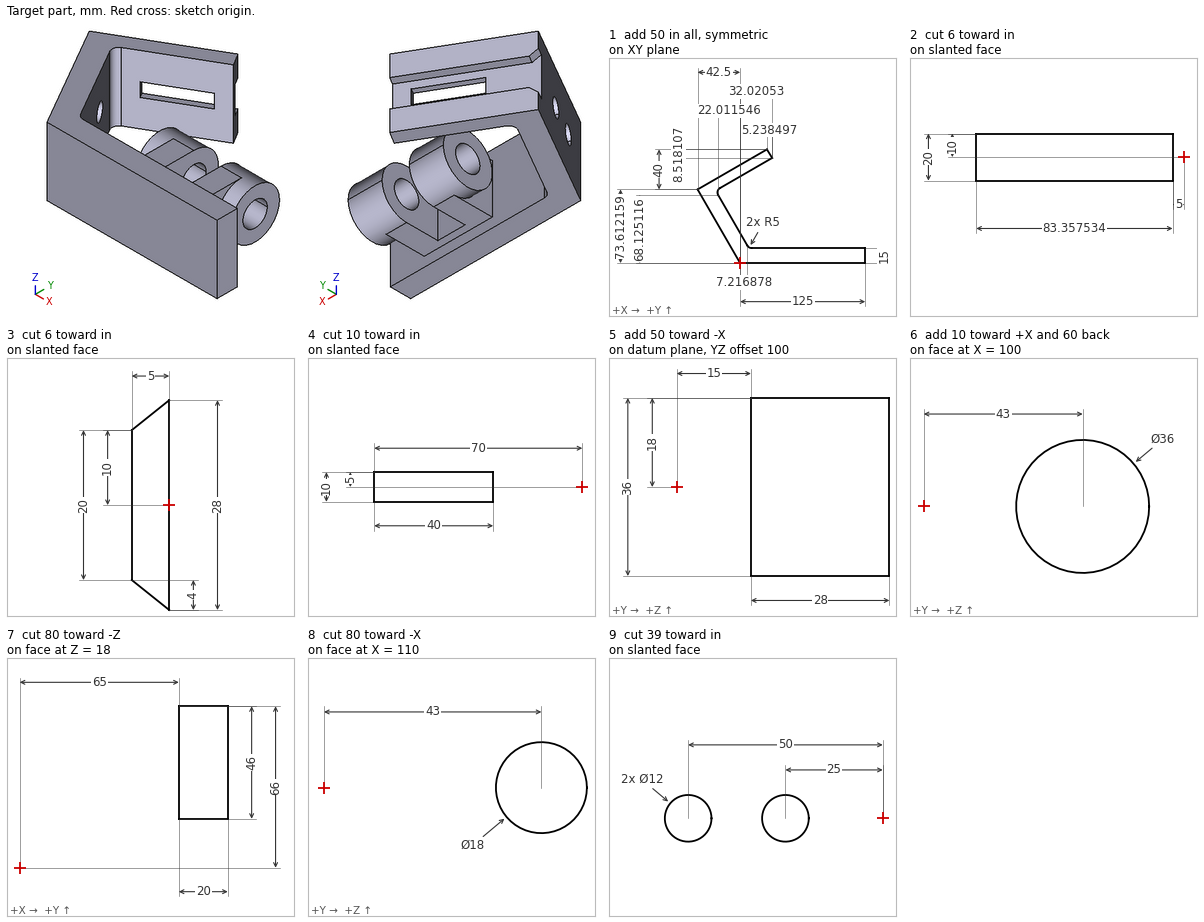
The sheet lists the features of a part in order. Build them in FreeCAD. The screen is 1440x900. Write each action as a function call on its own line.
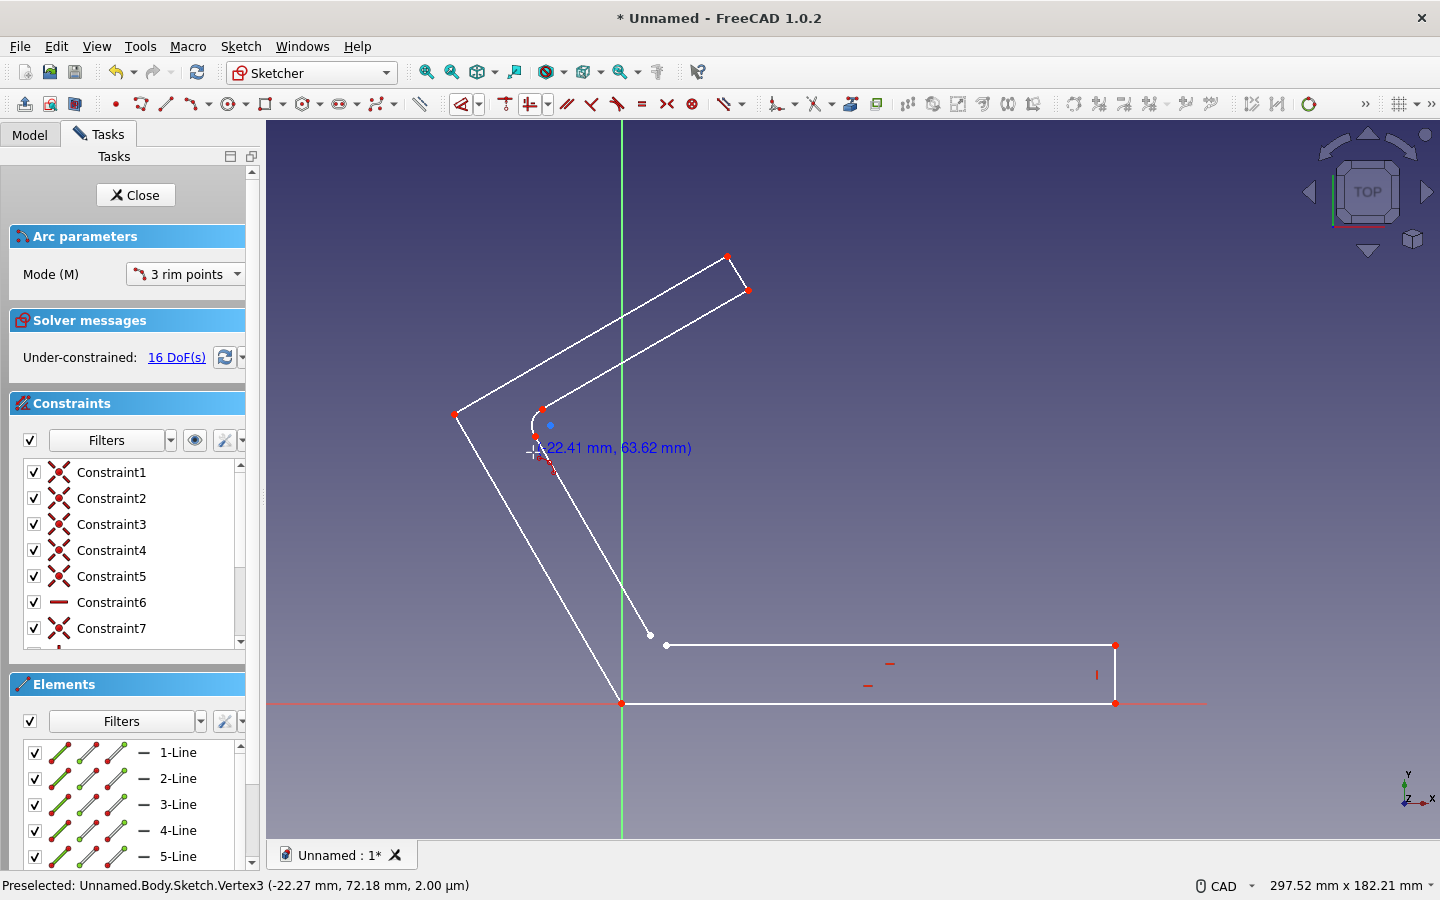
click(667, 645)
click(650, 635)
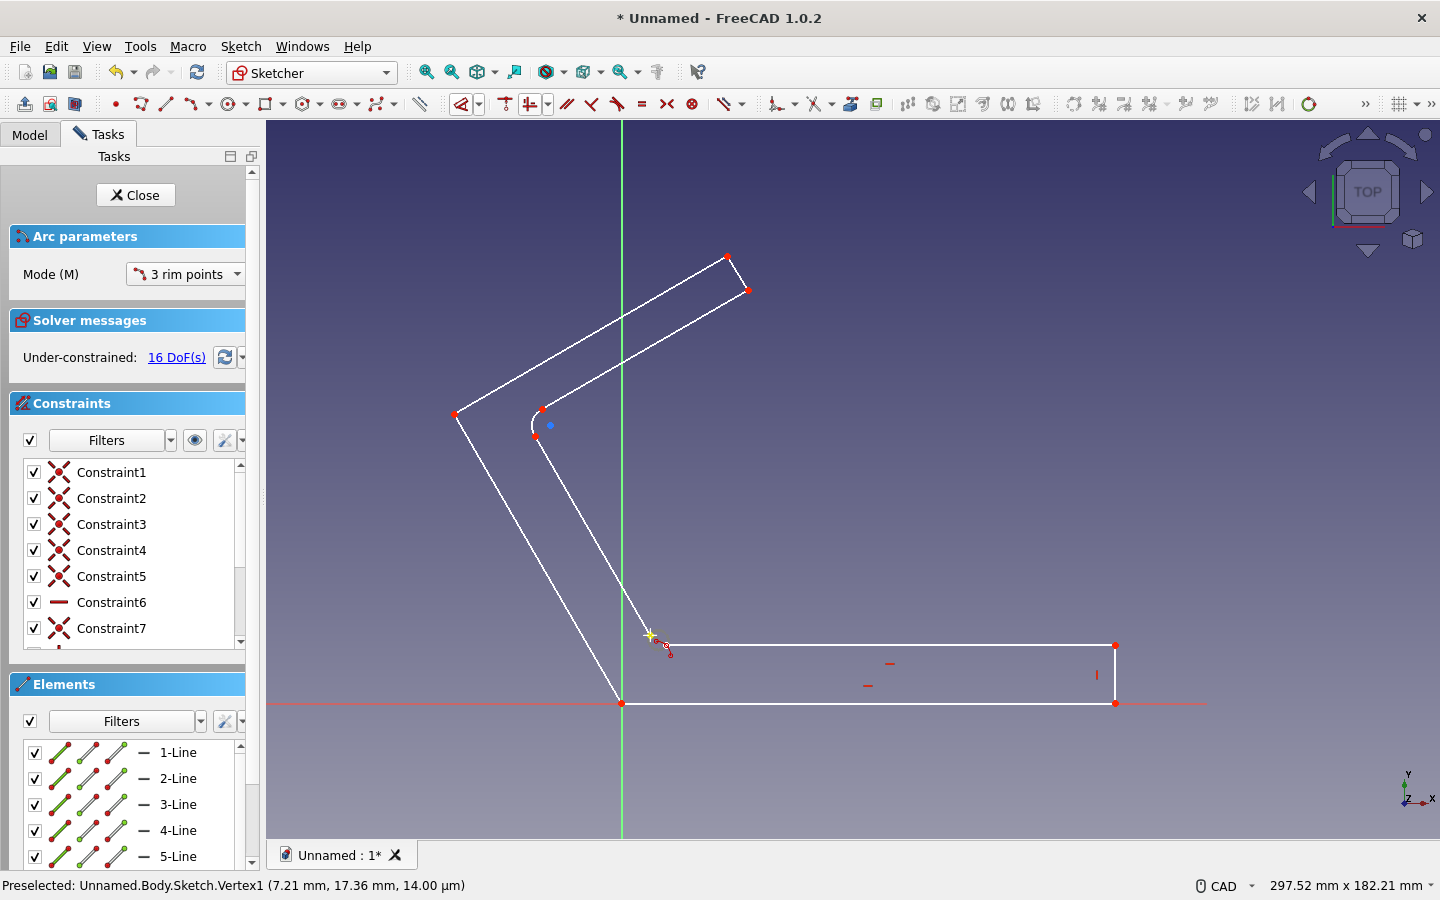
scroll(657, 642, up, 9)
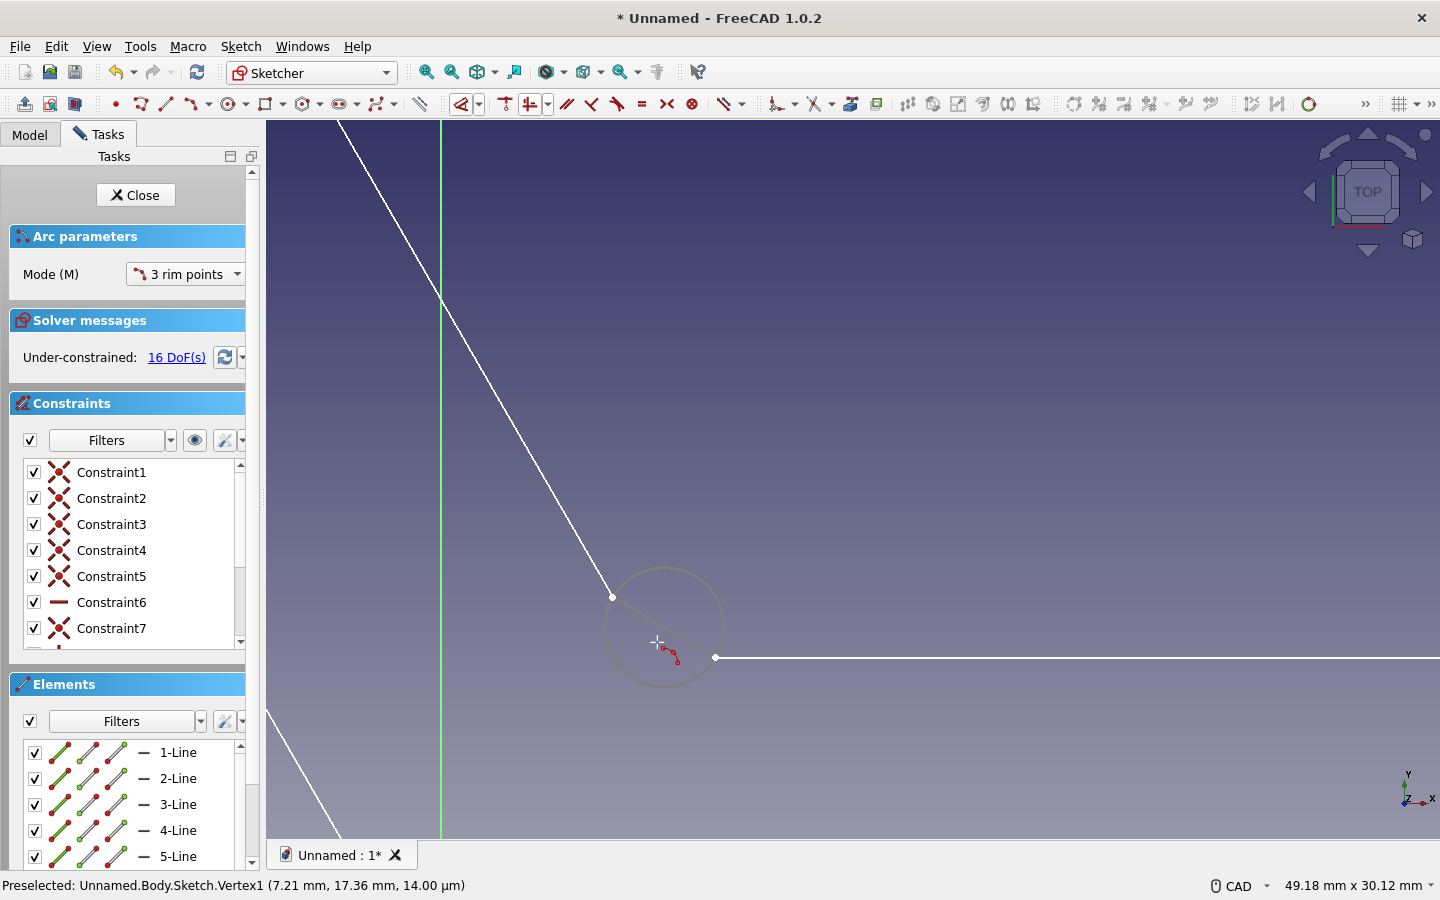
click(657, 637)
key(Escape)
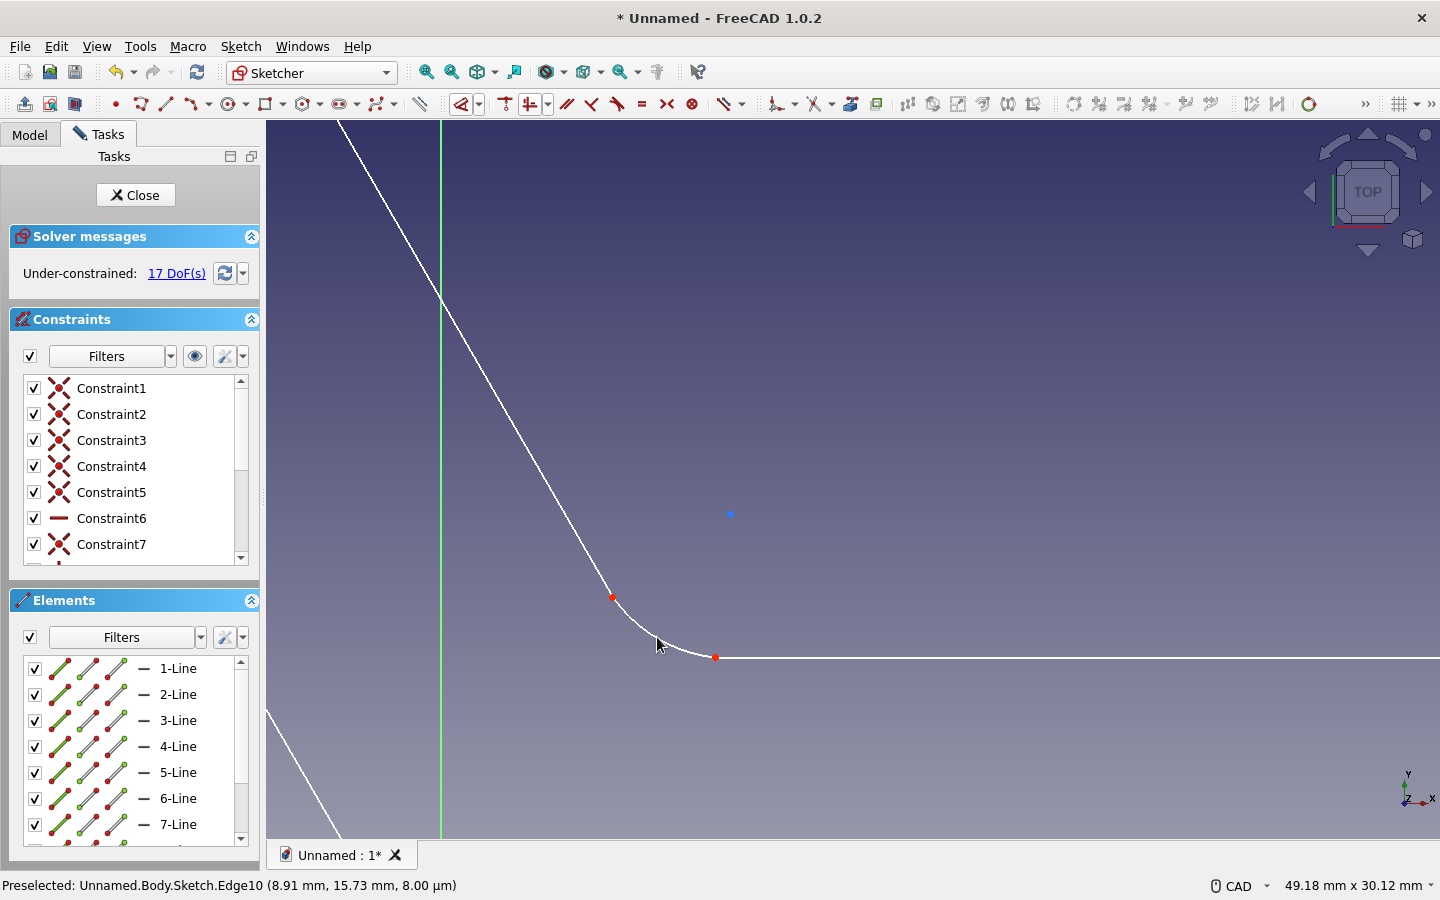
click(404, 236)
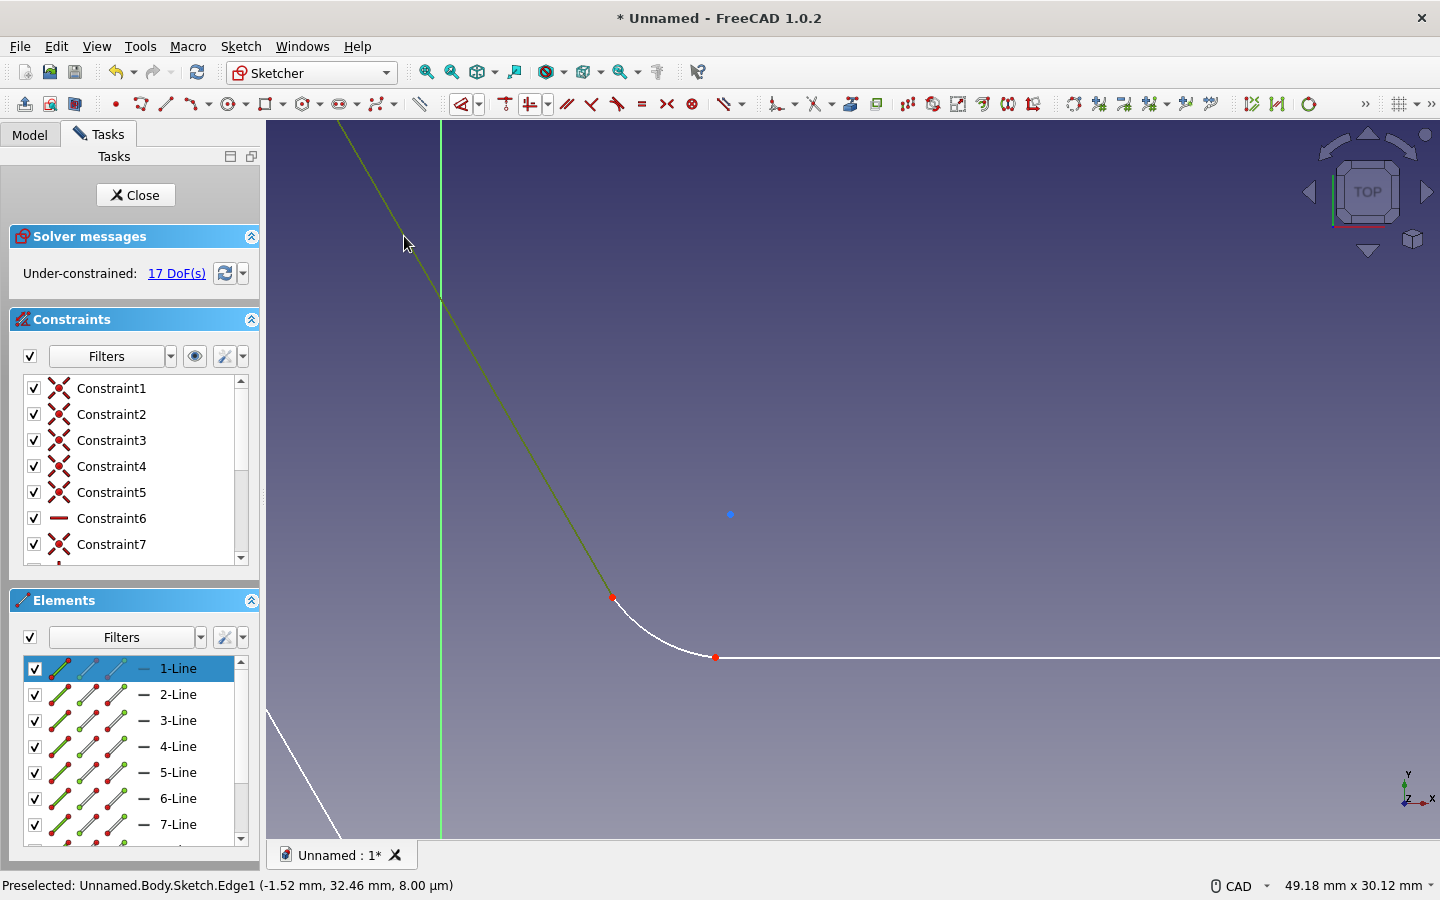
scroll(658, 643, down, 9)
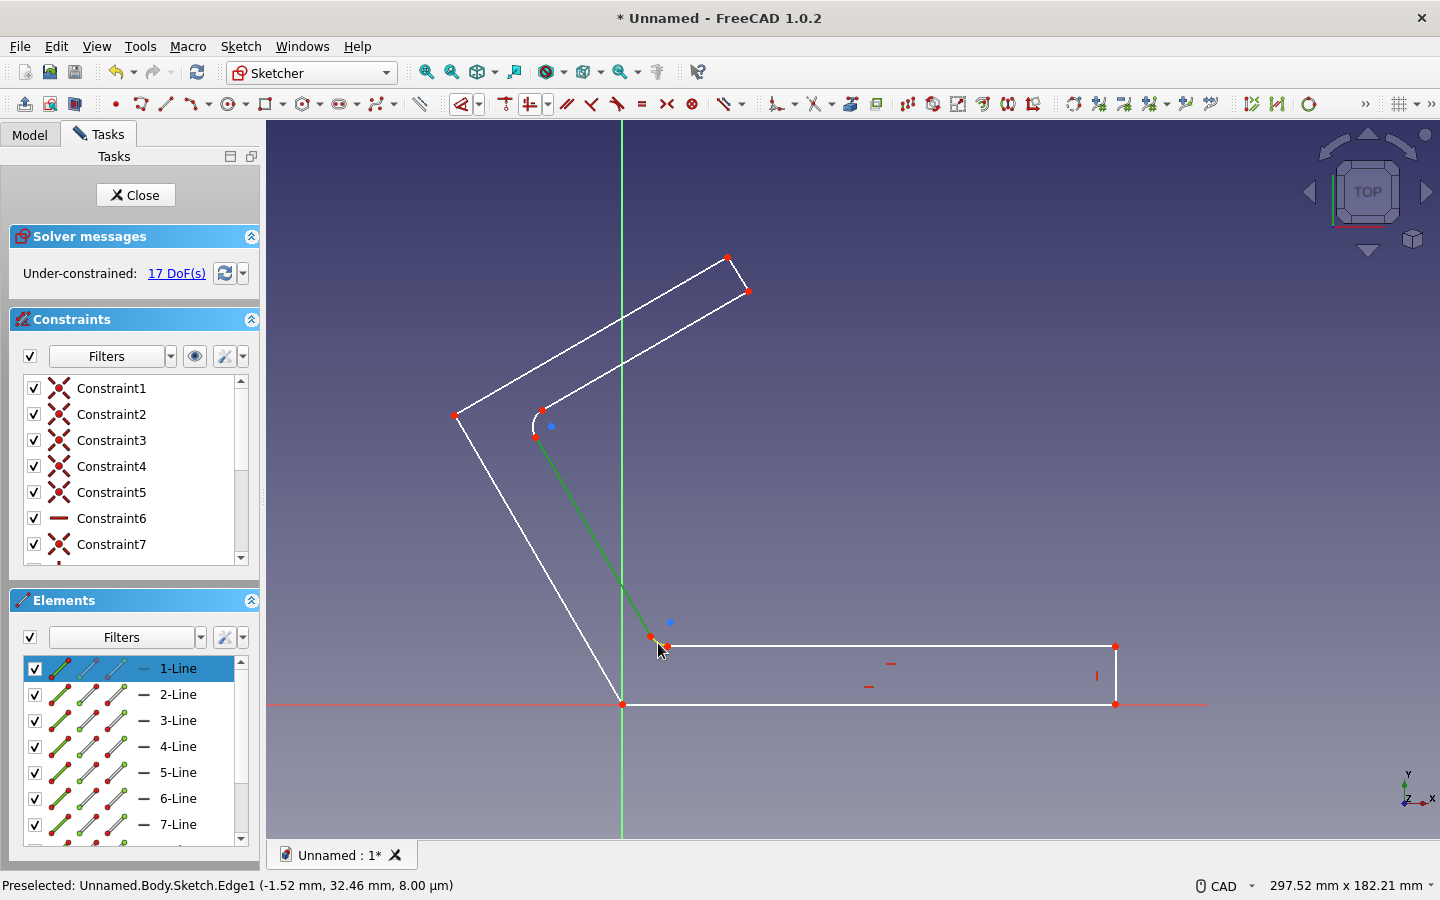
scroll(536, 416, up, 2)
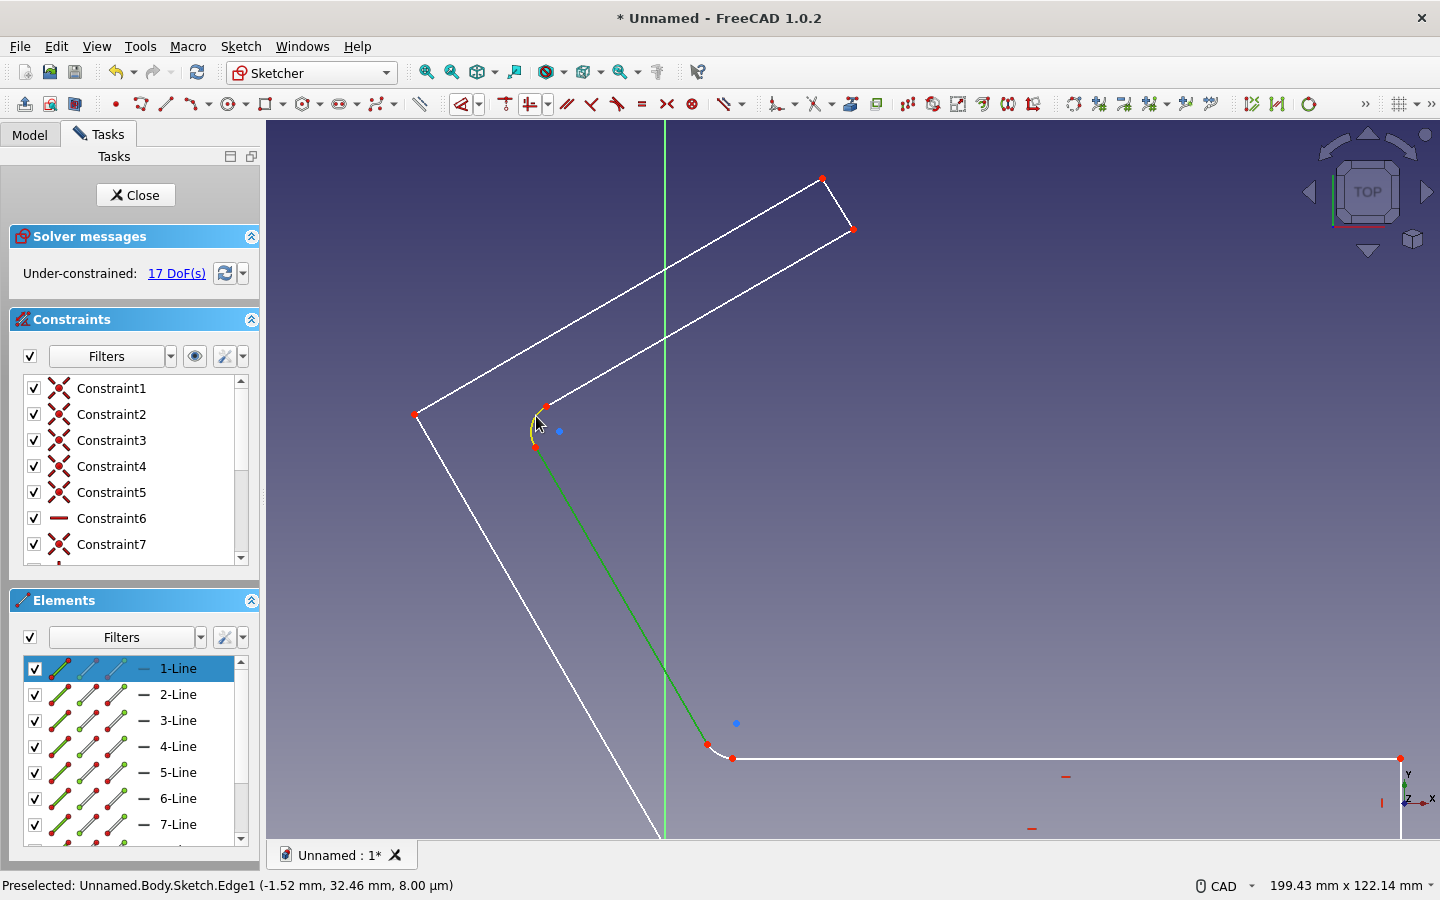
click(536, 416)